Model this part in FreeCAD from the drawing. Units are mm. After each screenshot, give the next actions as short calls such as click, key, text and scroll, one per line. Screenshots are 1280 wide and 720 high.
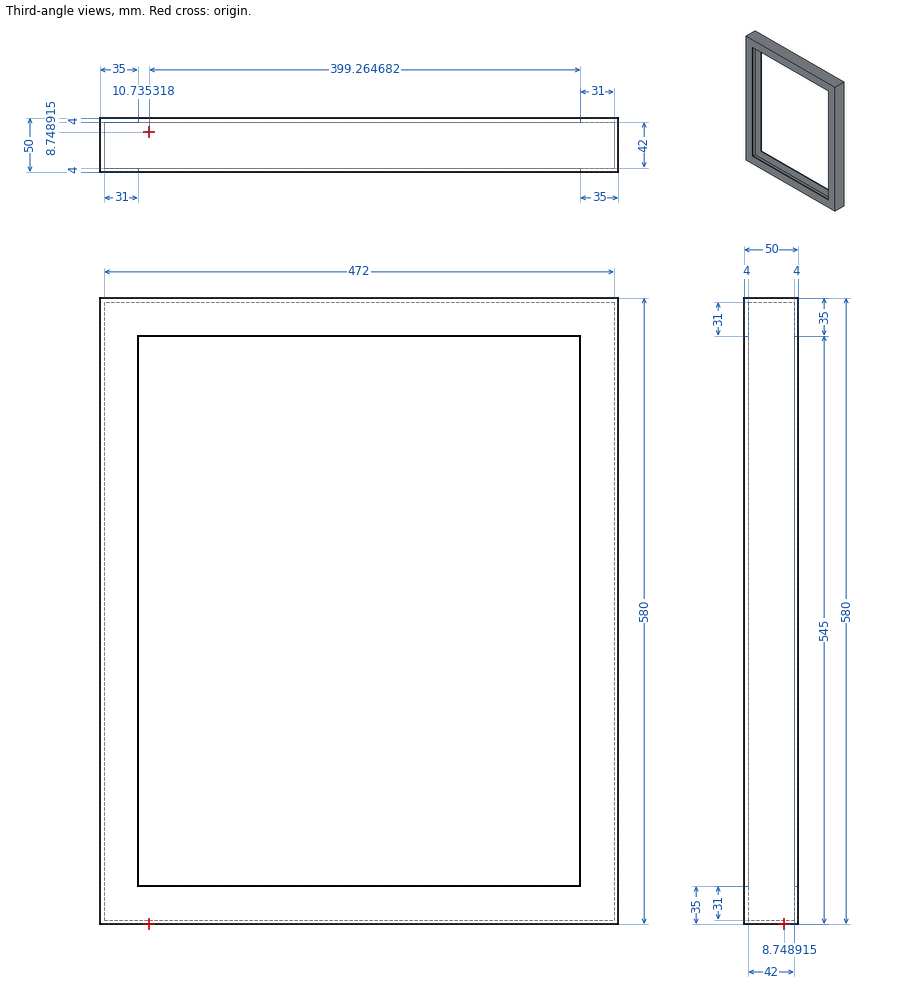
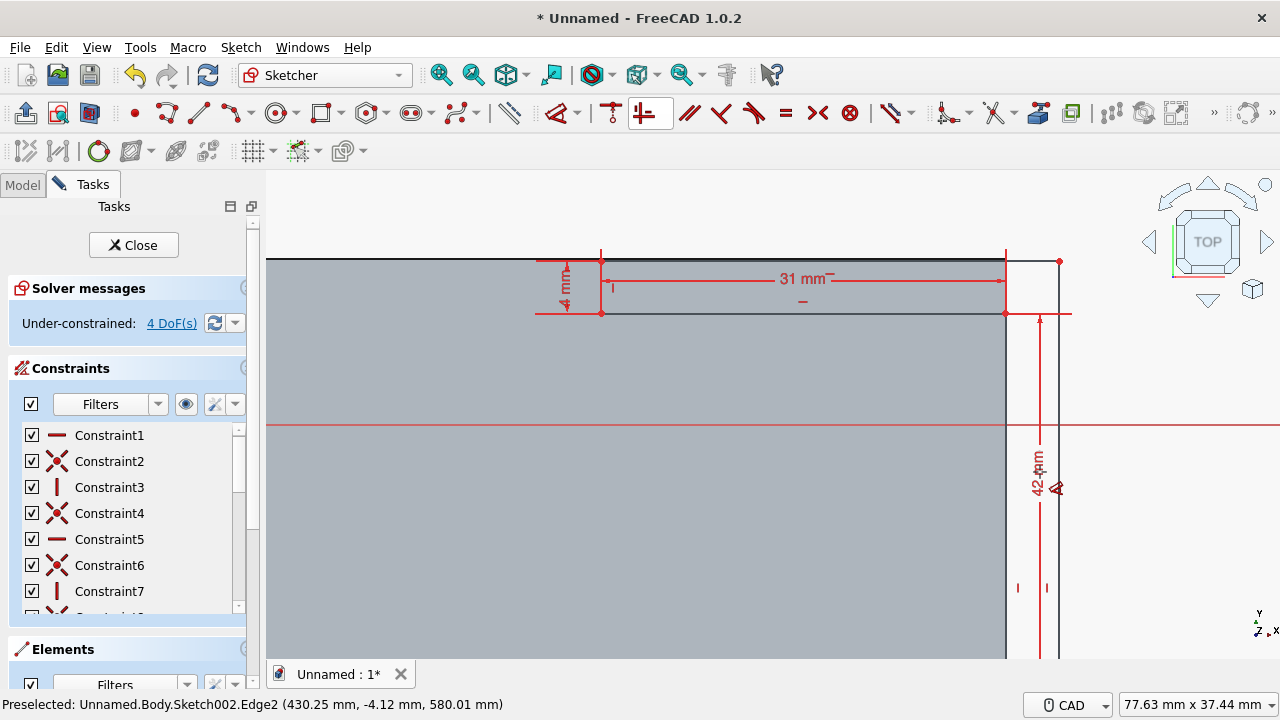
scroll(602, 275, down, 4)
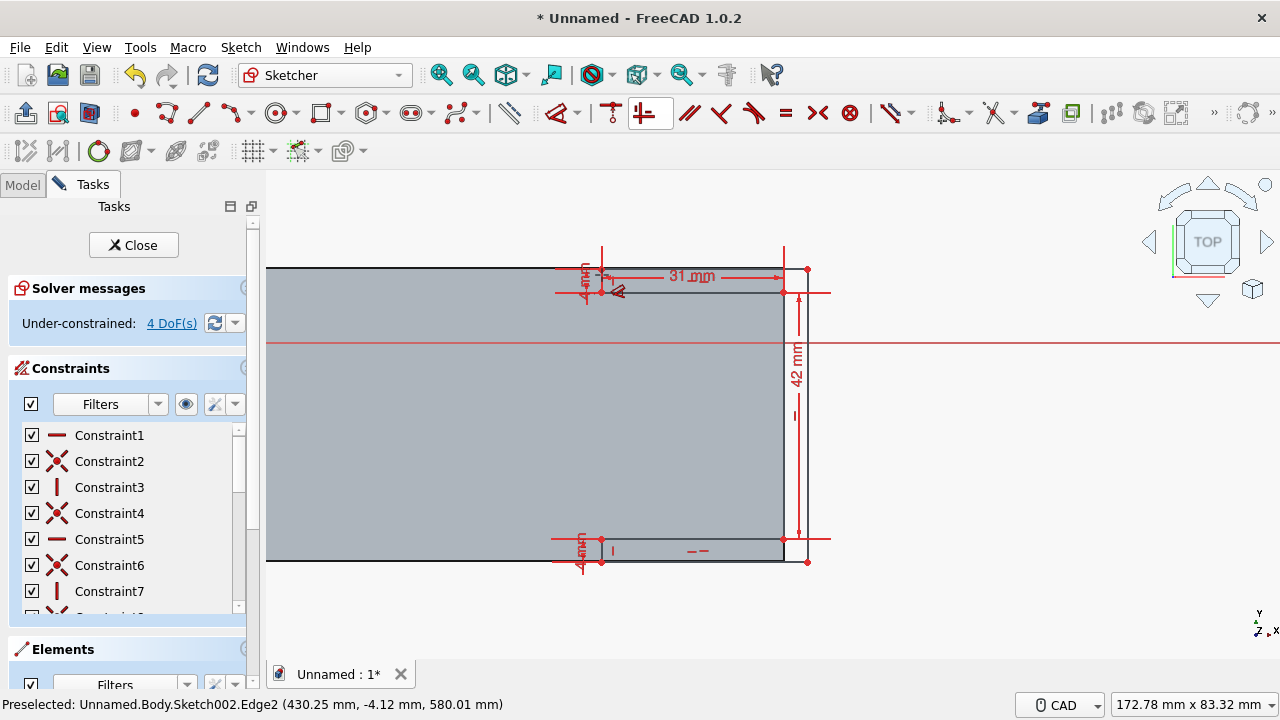
click(729, 539)
click(693, 505)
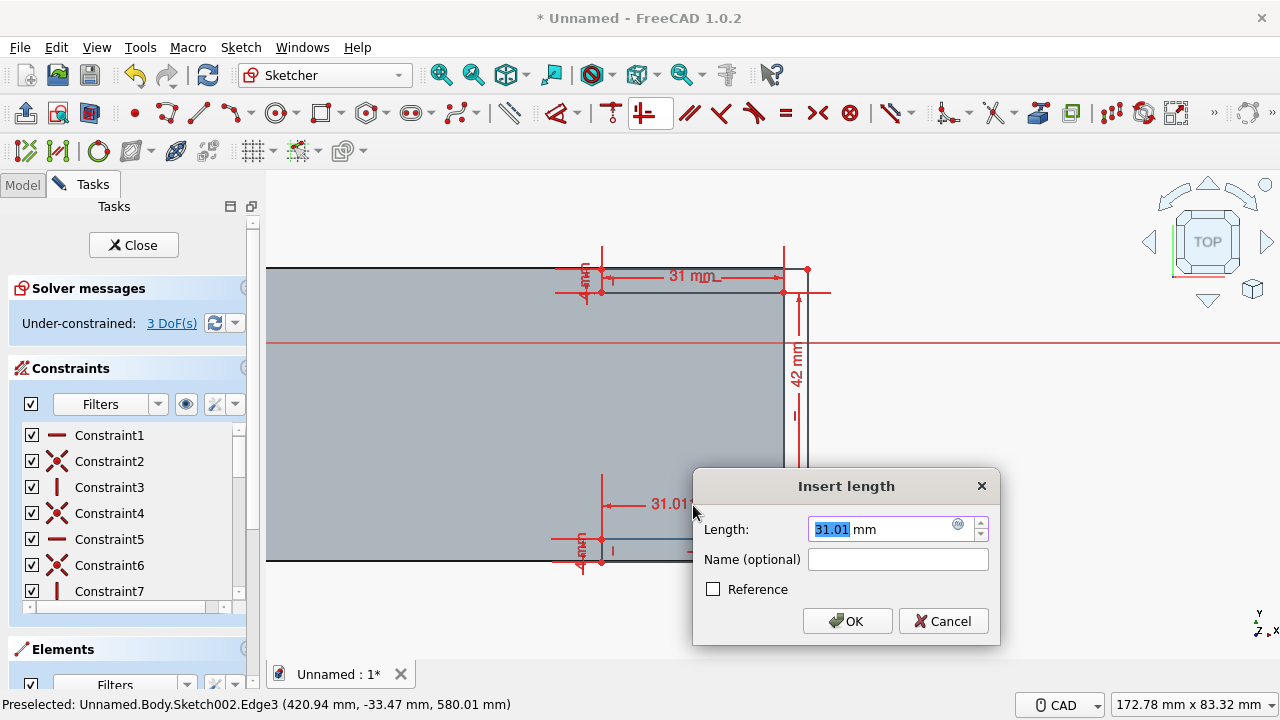
text(31)
key(Return)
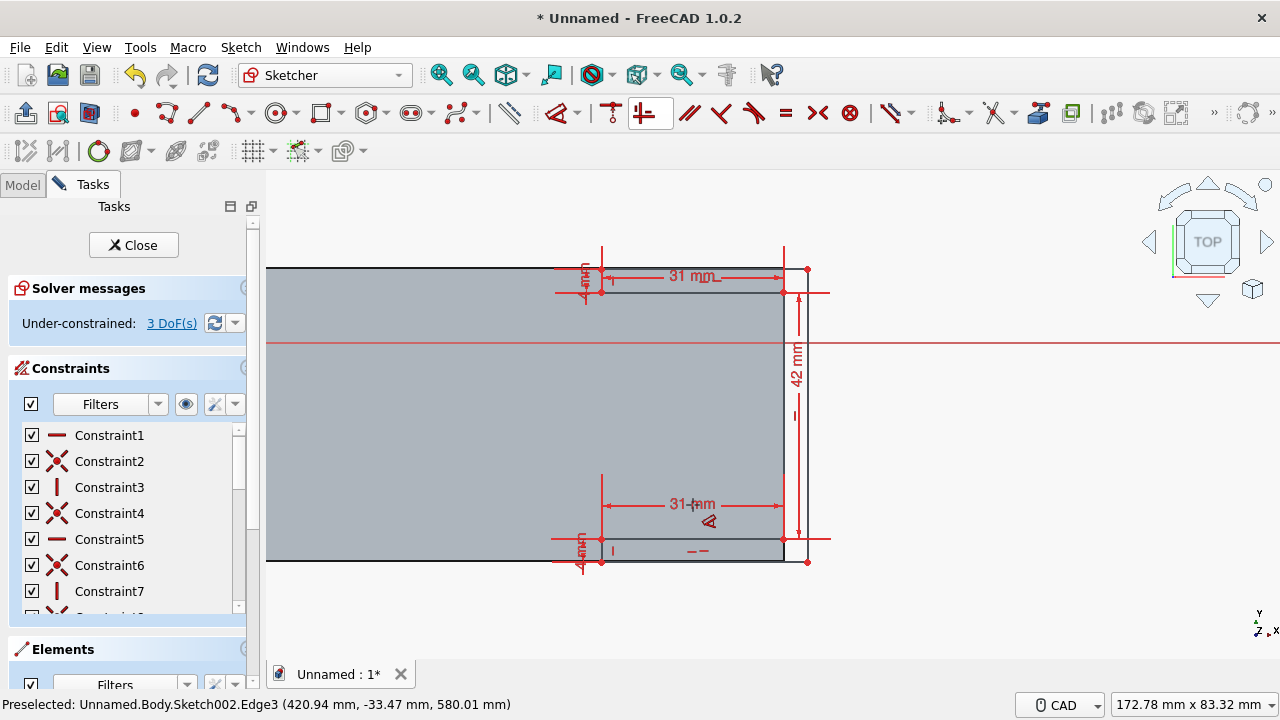
click(663, 562)
click(705, 596)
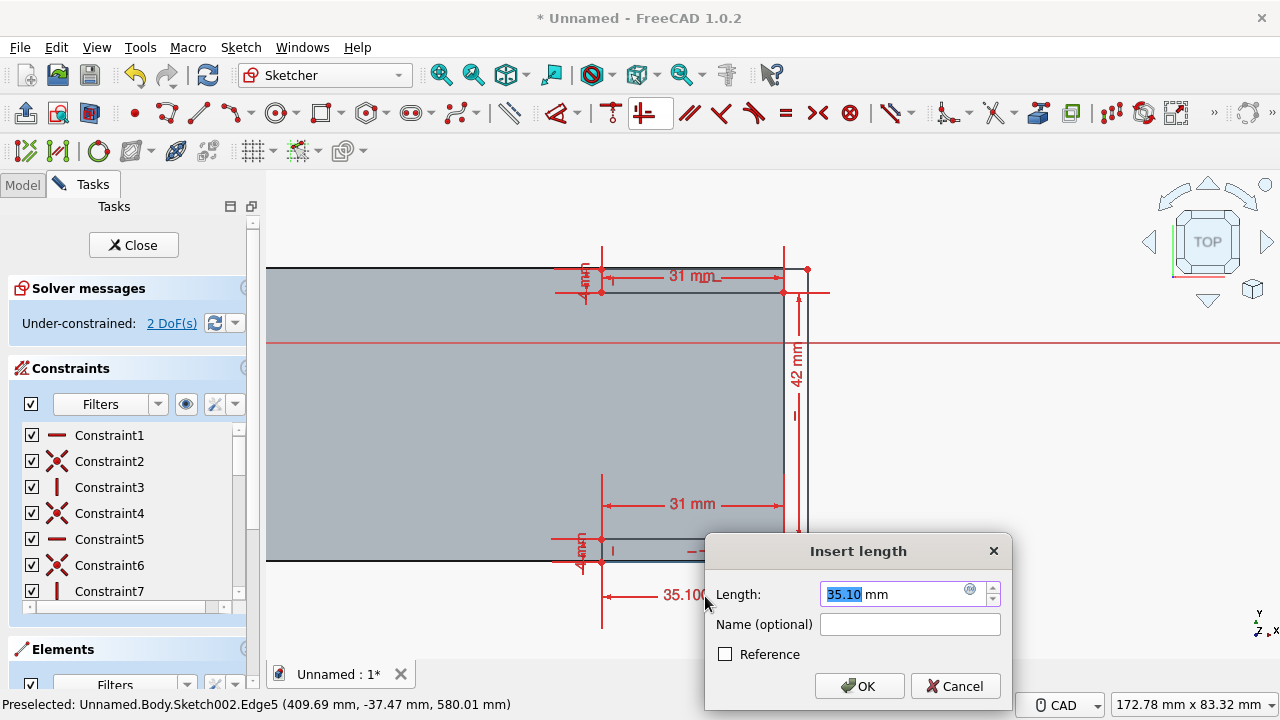
text(35)
key(Return)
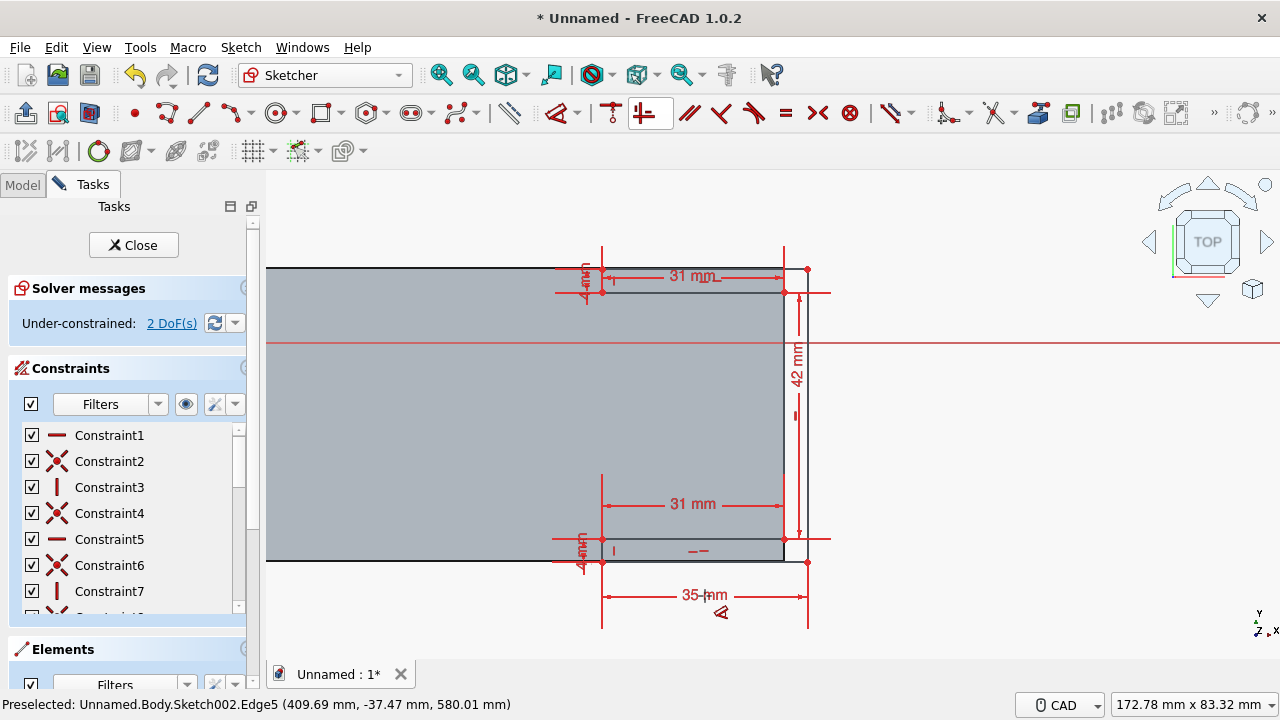
click(602, 293)
click(636, 318)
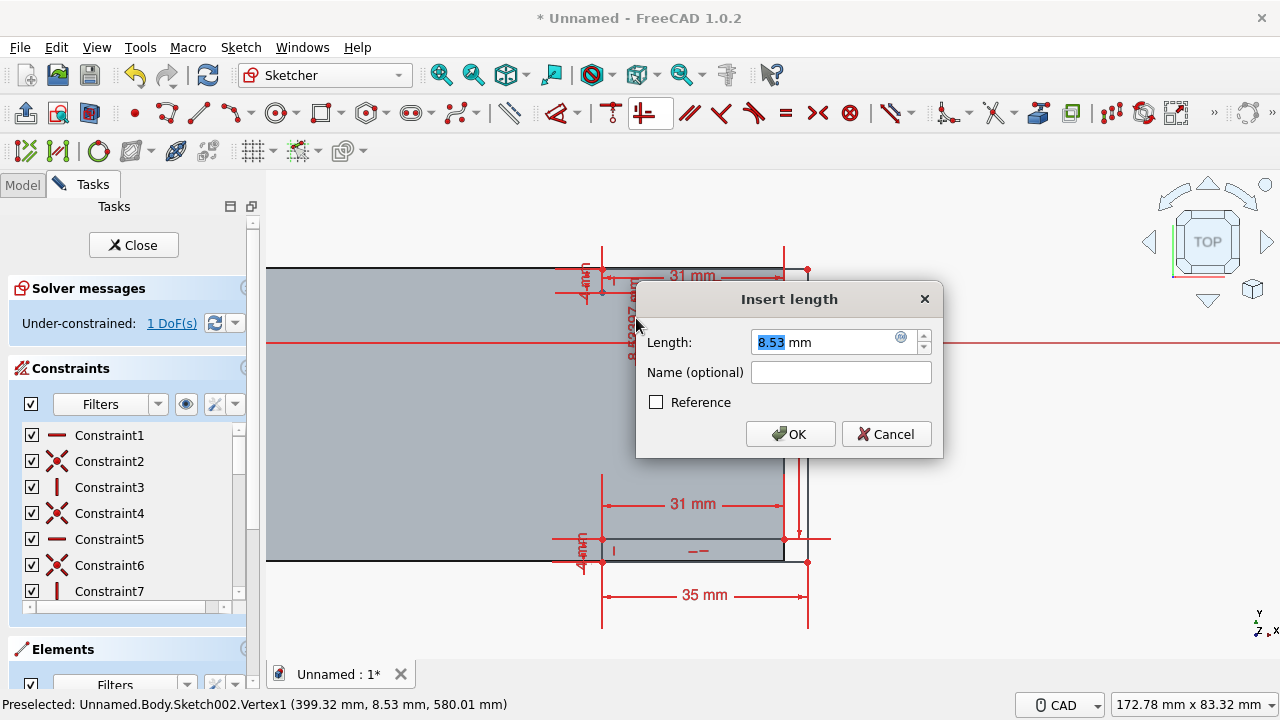
text(8.748915)
key(Return)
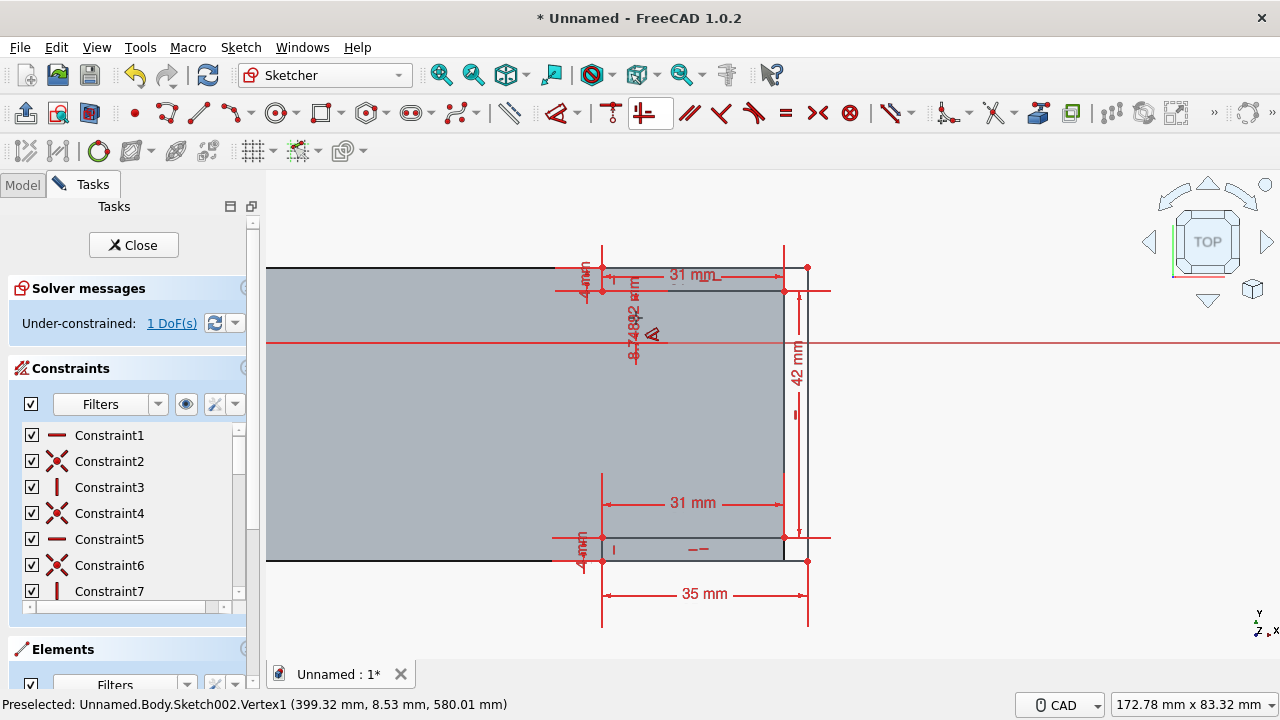
click(602, 291)
click(448, 257)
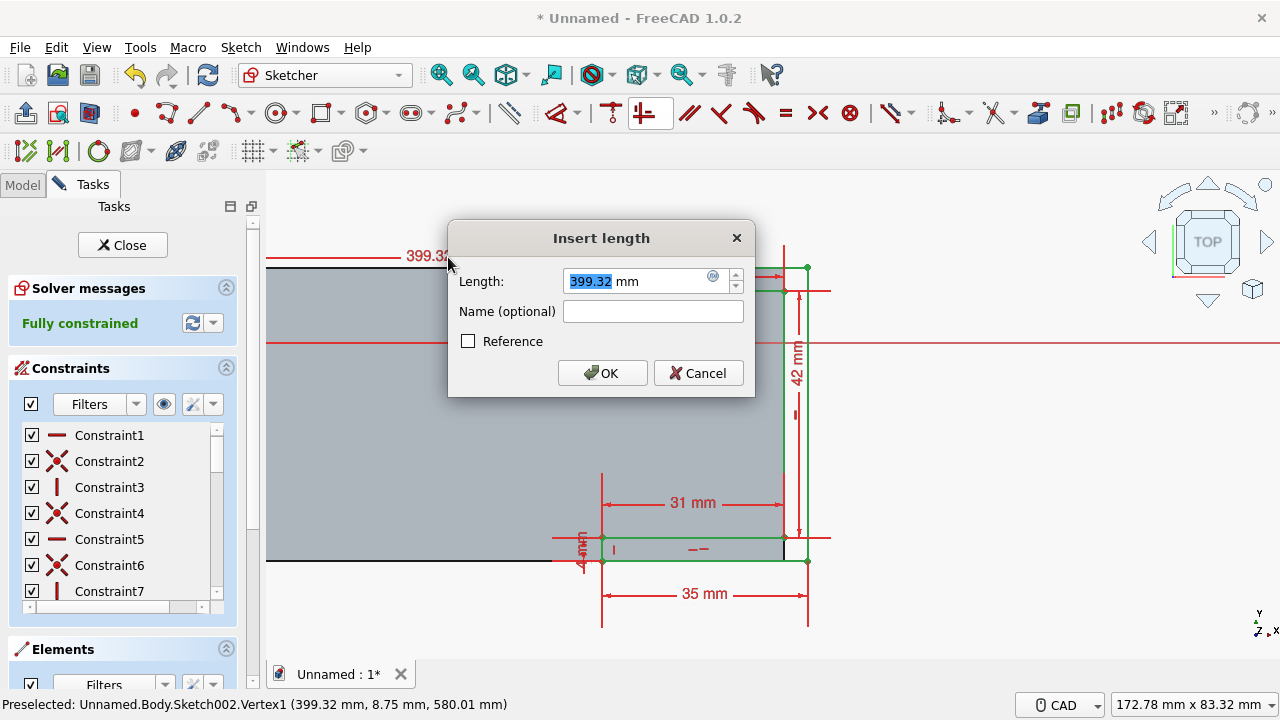
text(399.264682)
key(Return)
key(Escape)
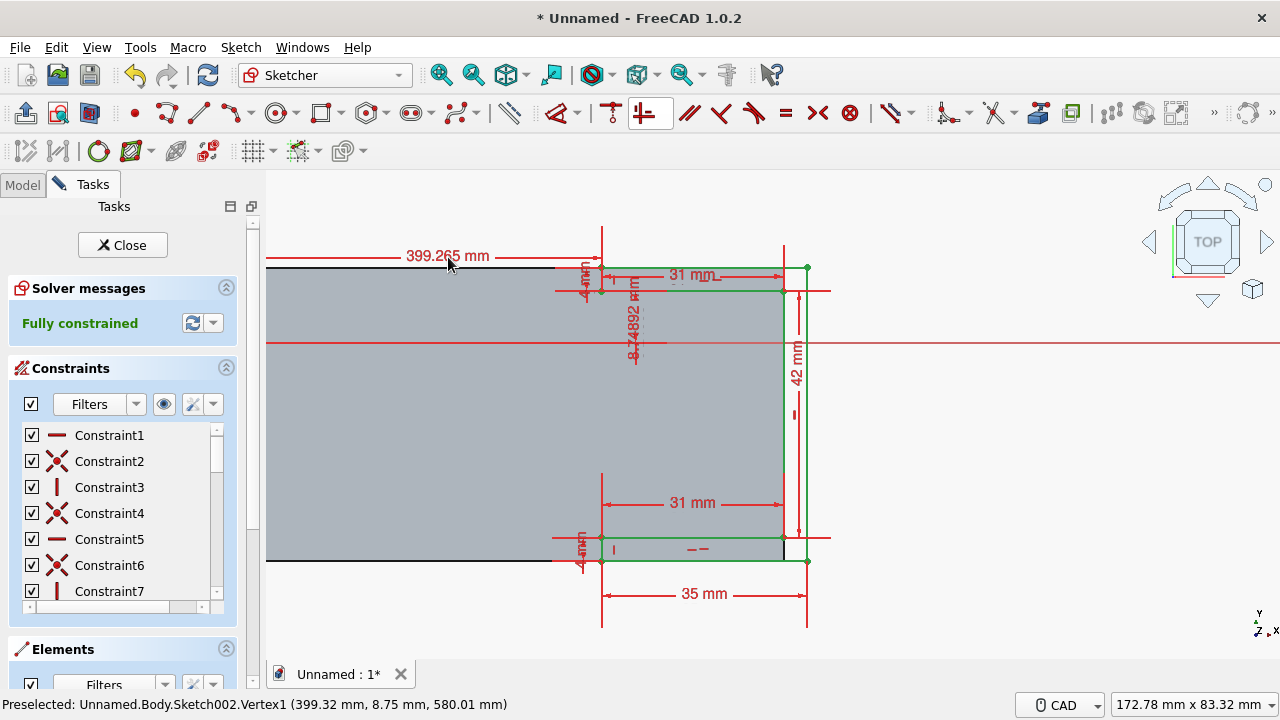
click(123, 245)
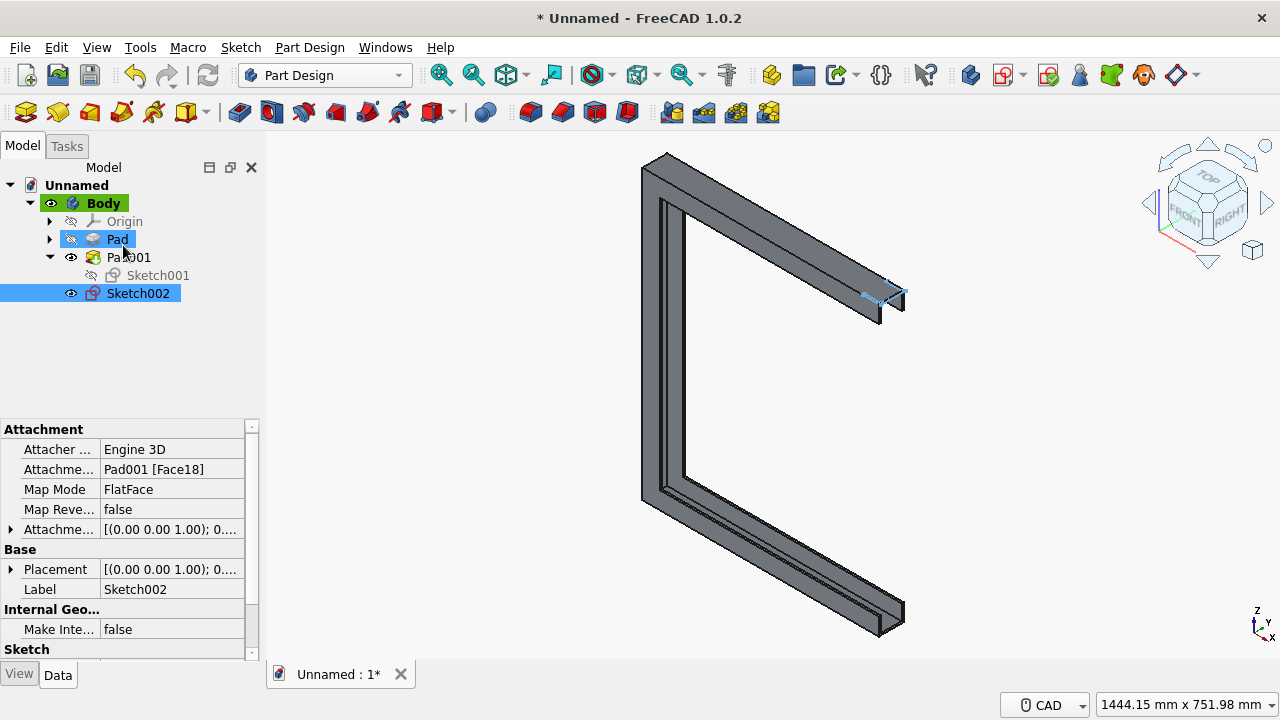
click(26, 112)